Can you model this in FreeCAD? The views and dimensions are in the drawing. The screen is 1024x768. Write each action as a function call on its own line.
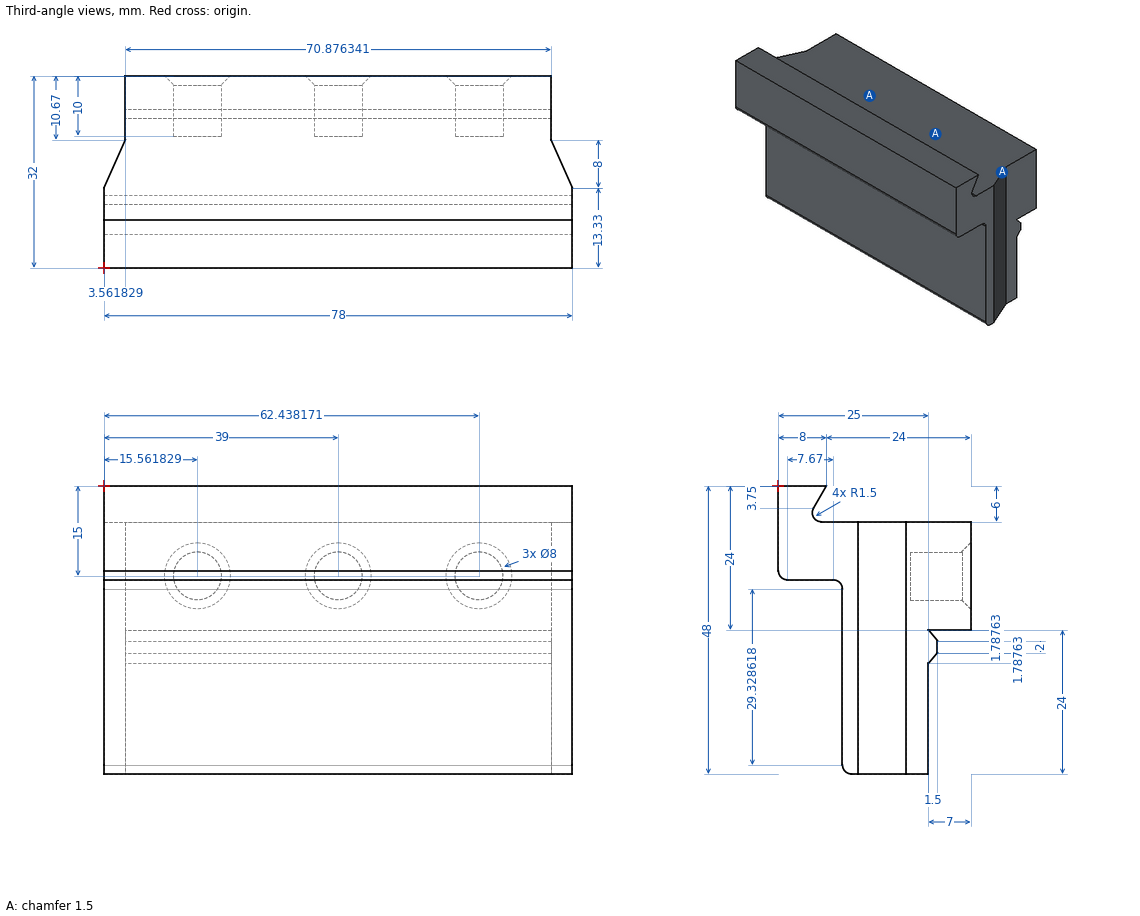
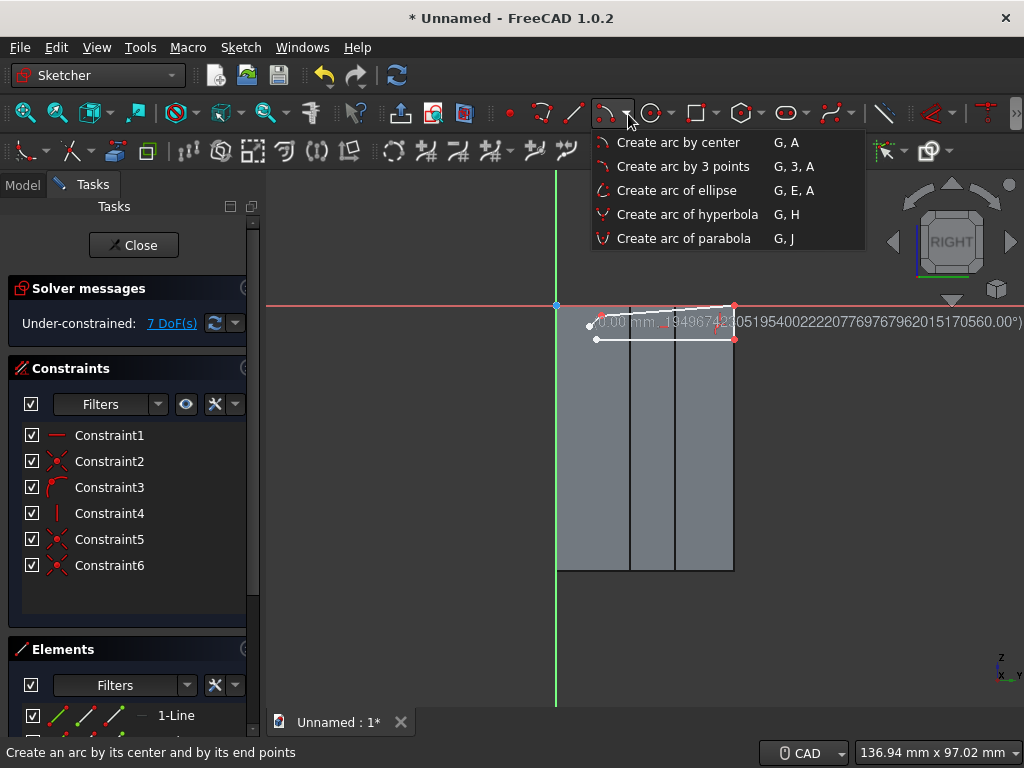
click(728, 166)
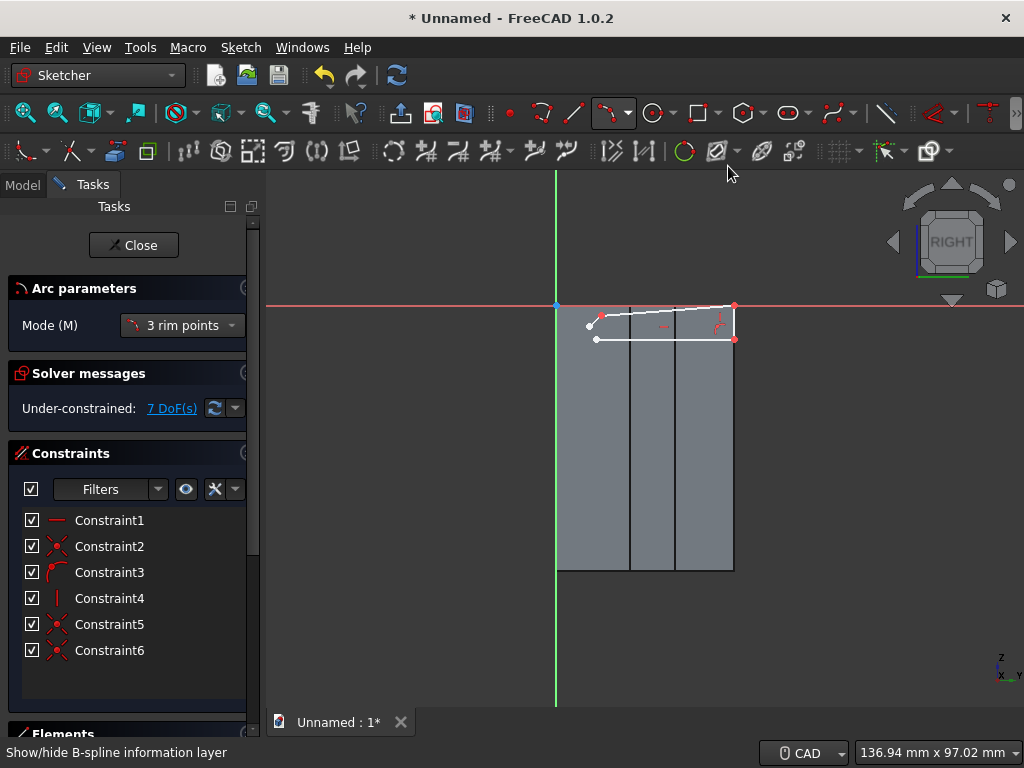
scroll(589, 326, up, 2)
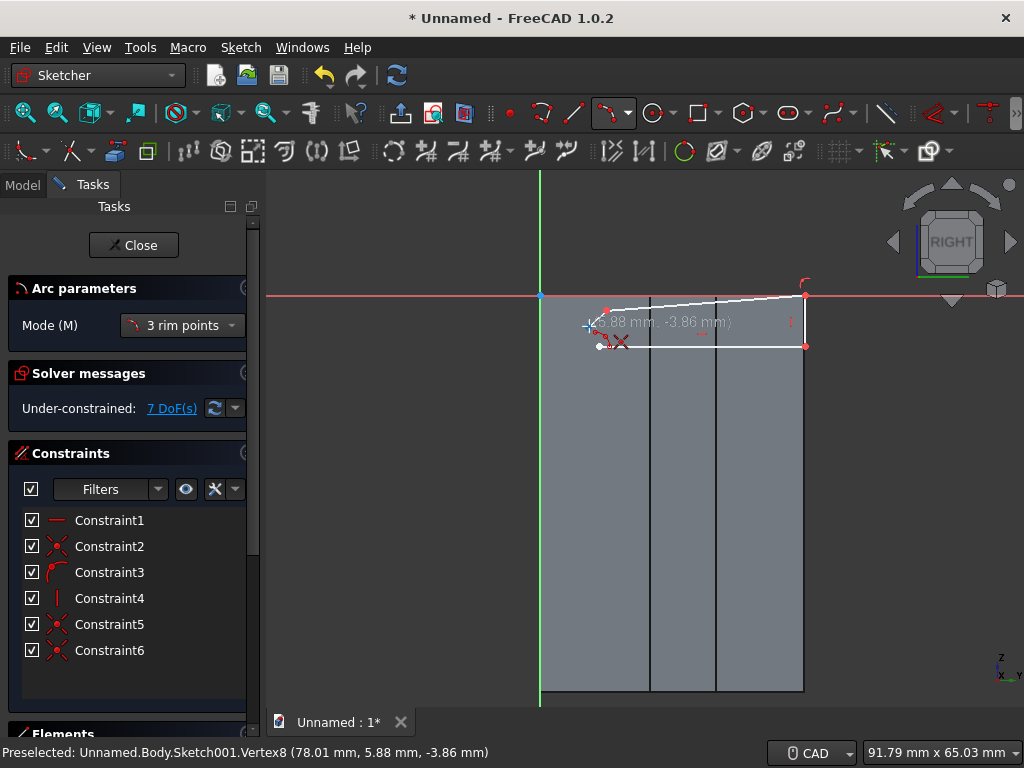
click(589, 327)
click(599, 347)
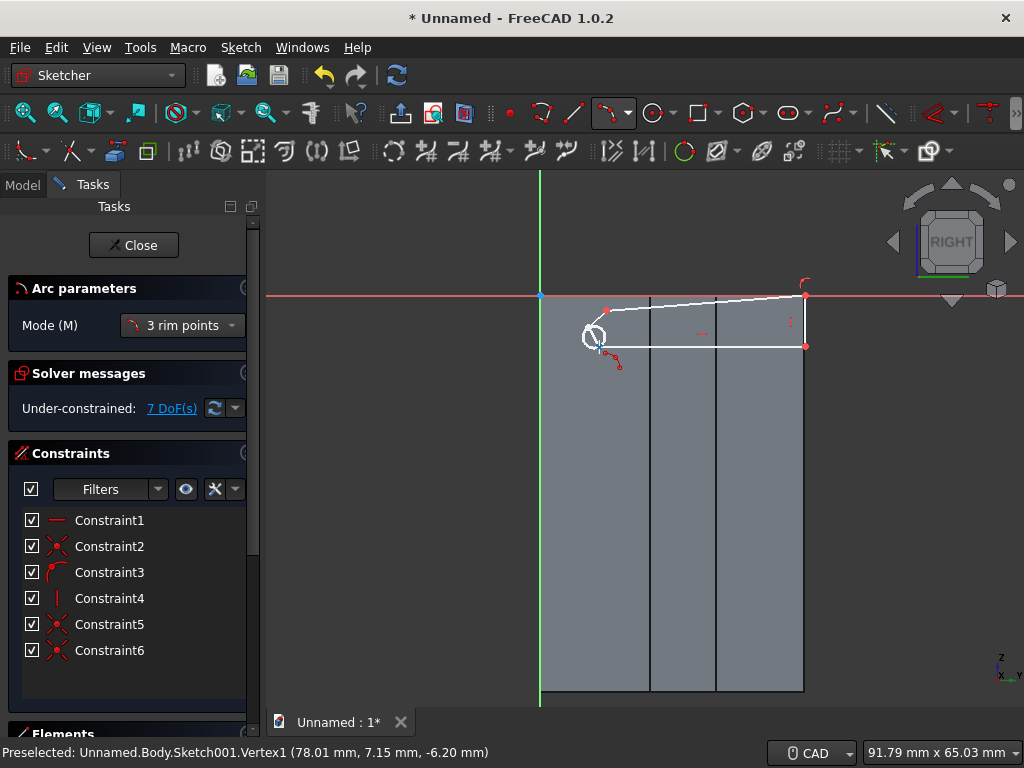
scroll(588, 339, up, 5)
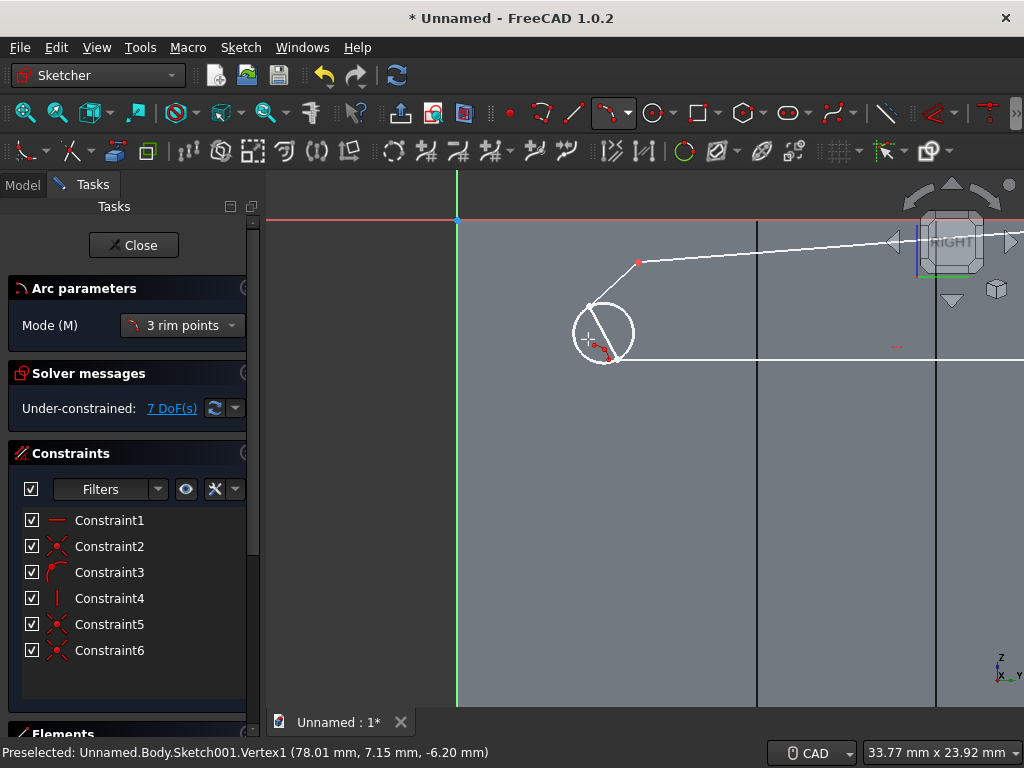
click(588, 338)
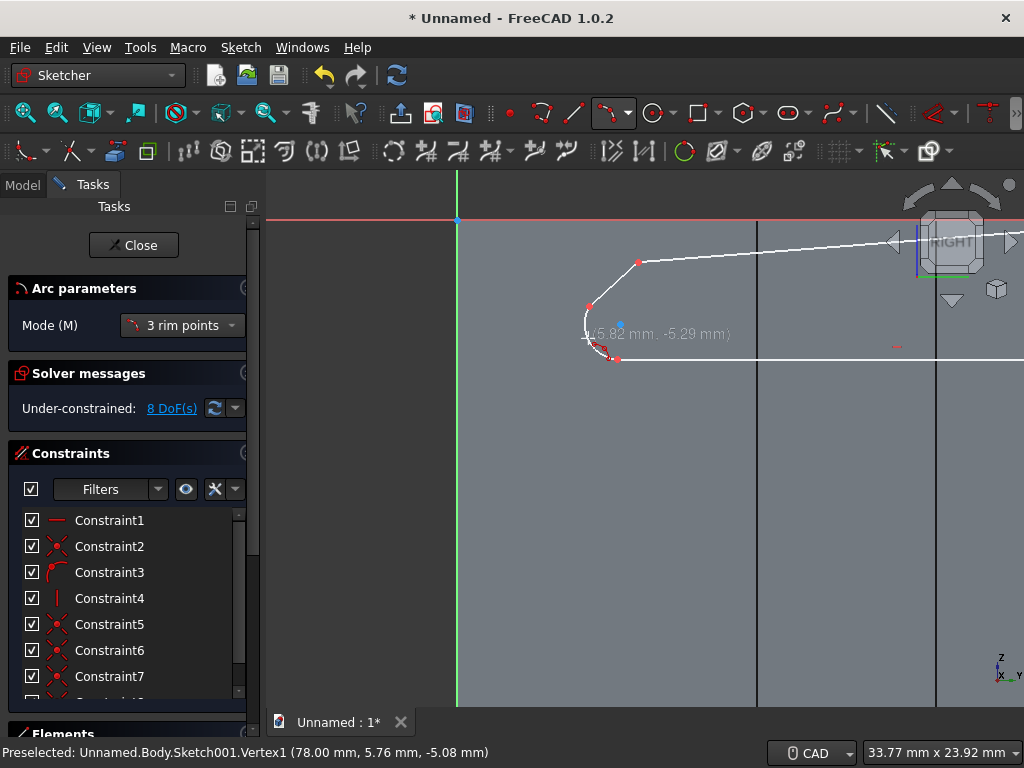
click(542, 114)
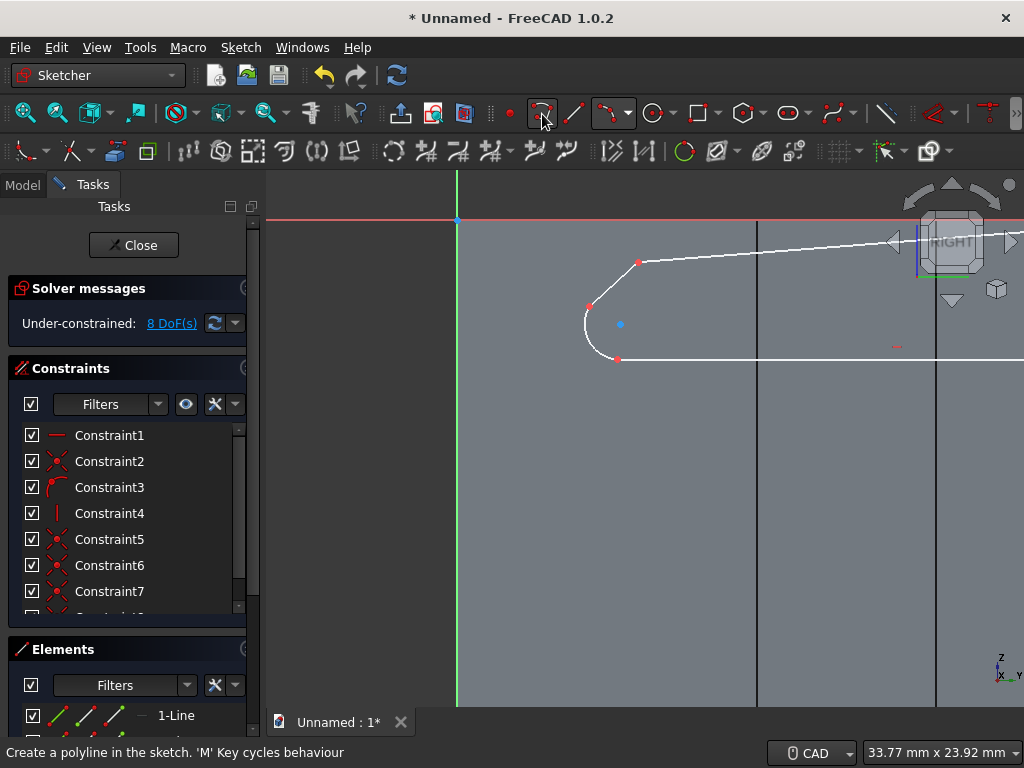
scroll(473, 300, down, 6)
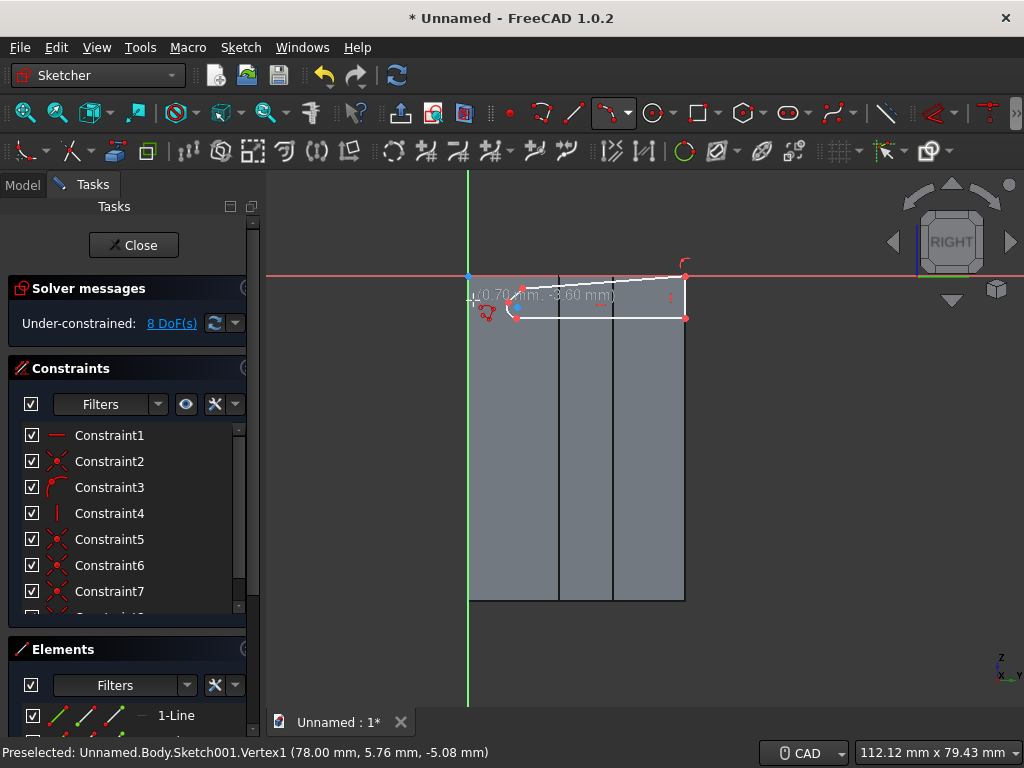
click(638, 438)
click(648, 450)
click(648, 464)
click(638, 476)
click(638, 601)
click(685, 601)
click(685, 438)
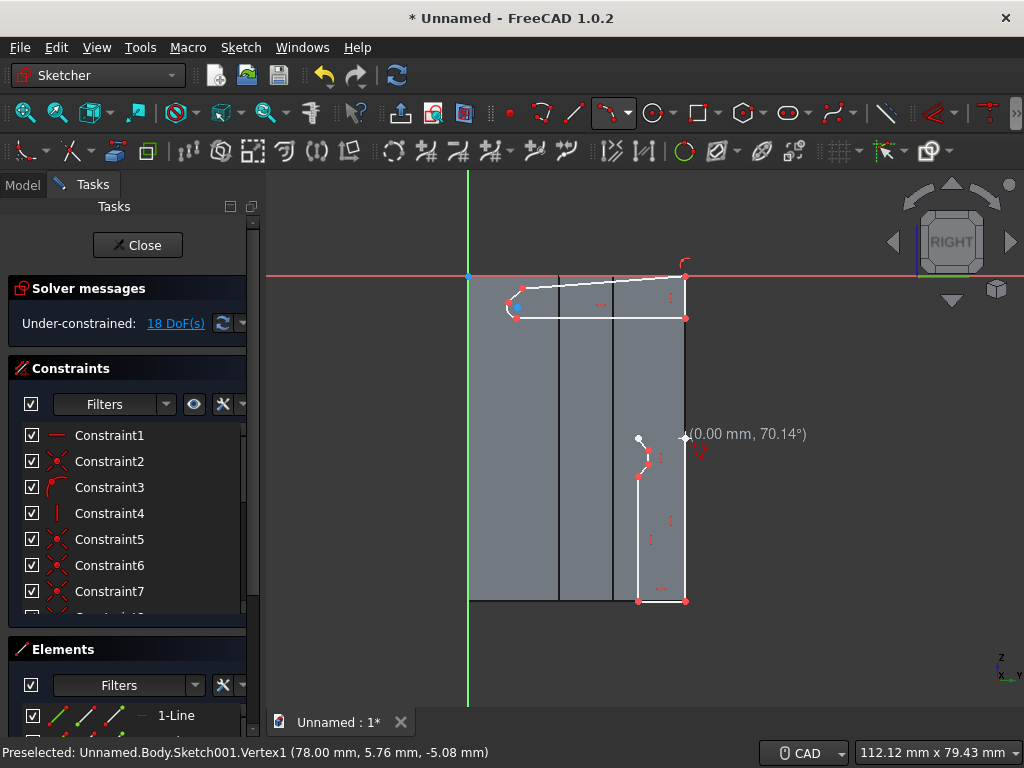
scroll(638, 438, up, 4)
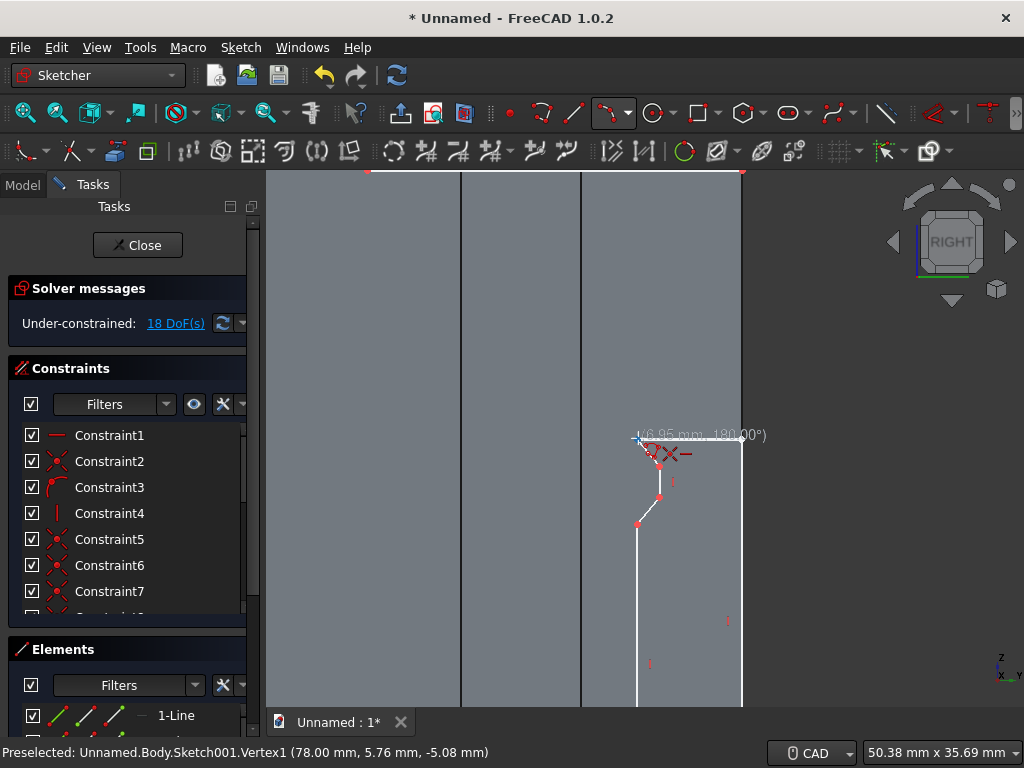
click(637, 440)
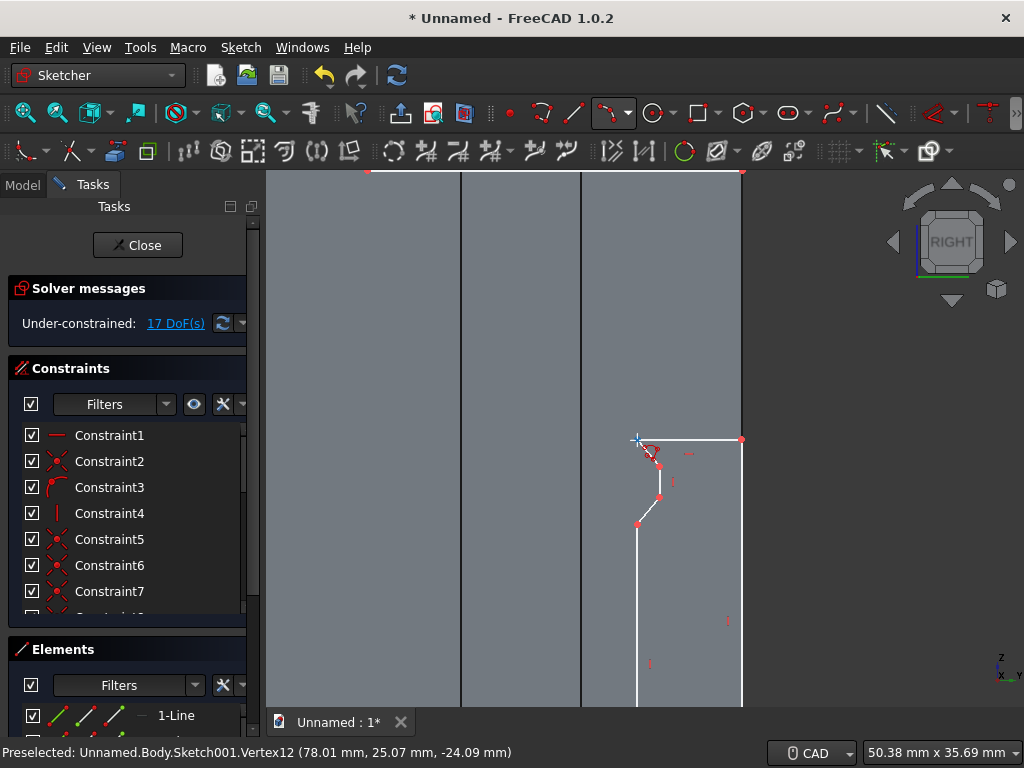
click(574, 114)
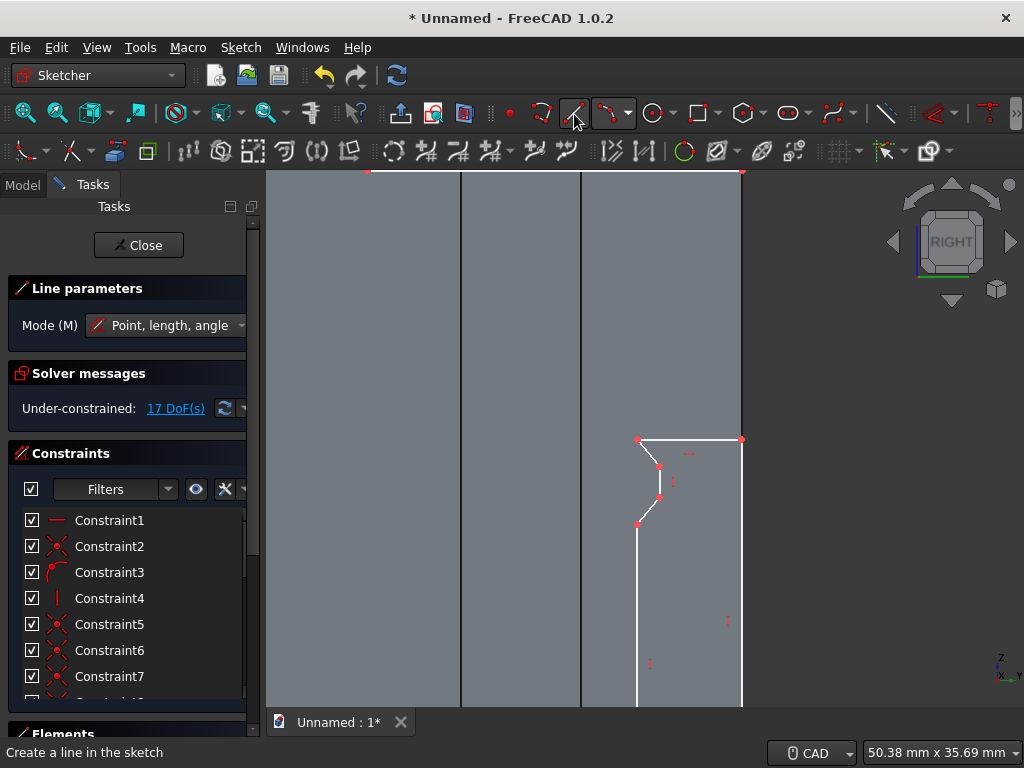
scroll(638, 439, down, 4)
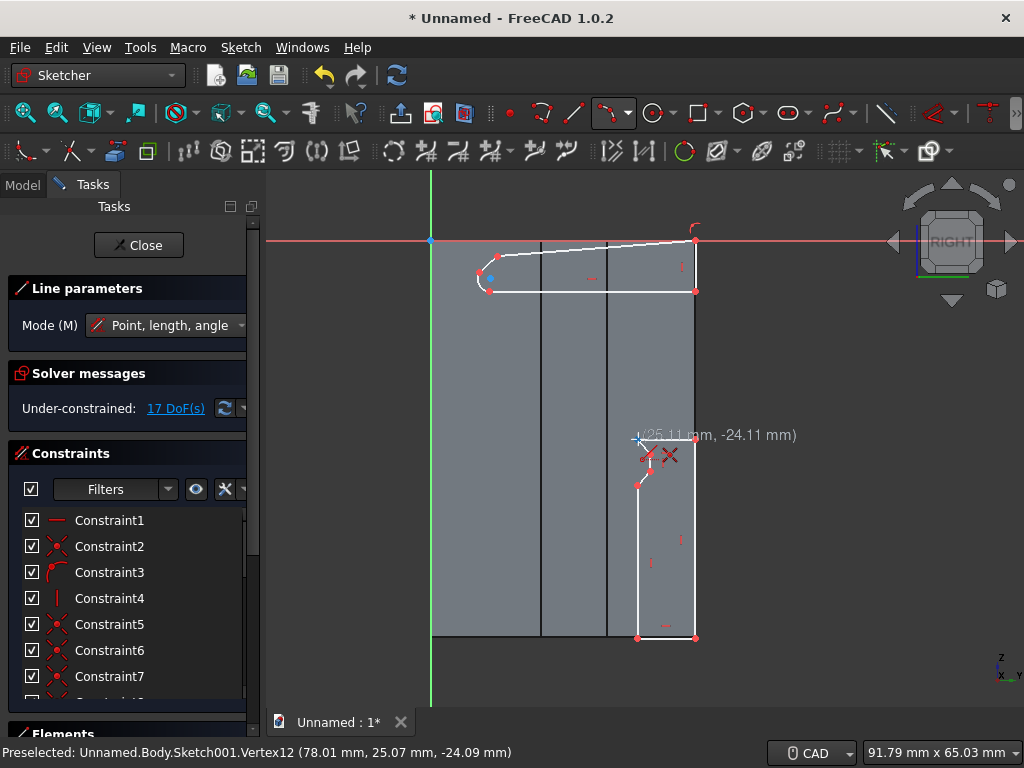
click(541, 591)
click(541, 393)